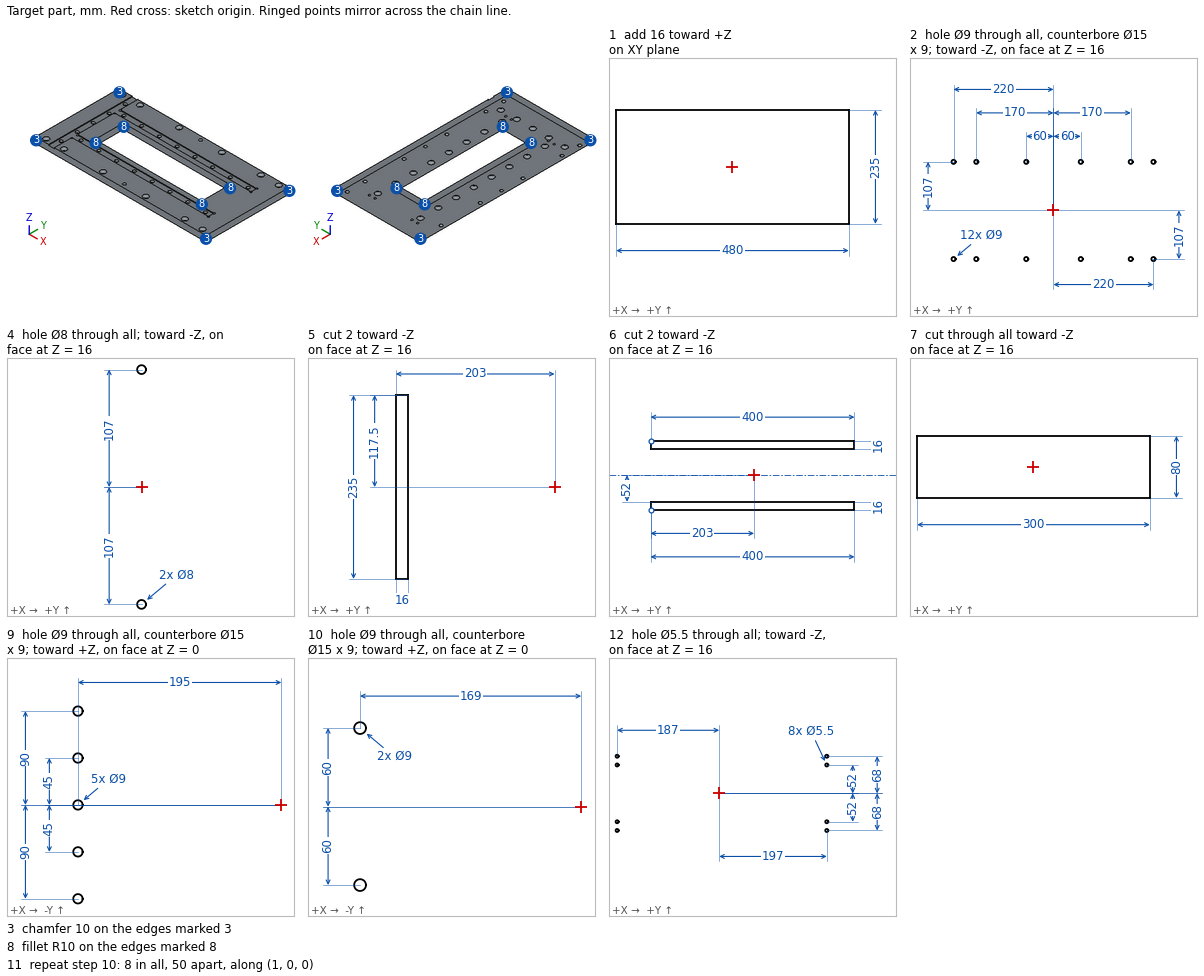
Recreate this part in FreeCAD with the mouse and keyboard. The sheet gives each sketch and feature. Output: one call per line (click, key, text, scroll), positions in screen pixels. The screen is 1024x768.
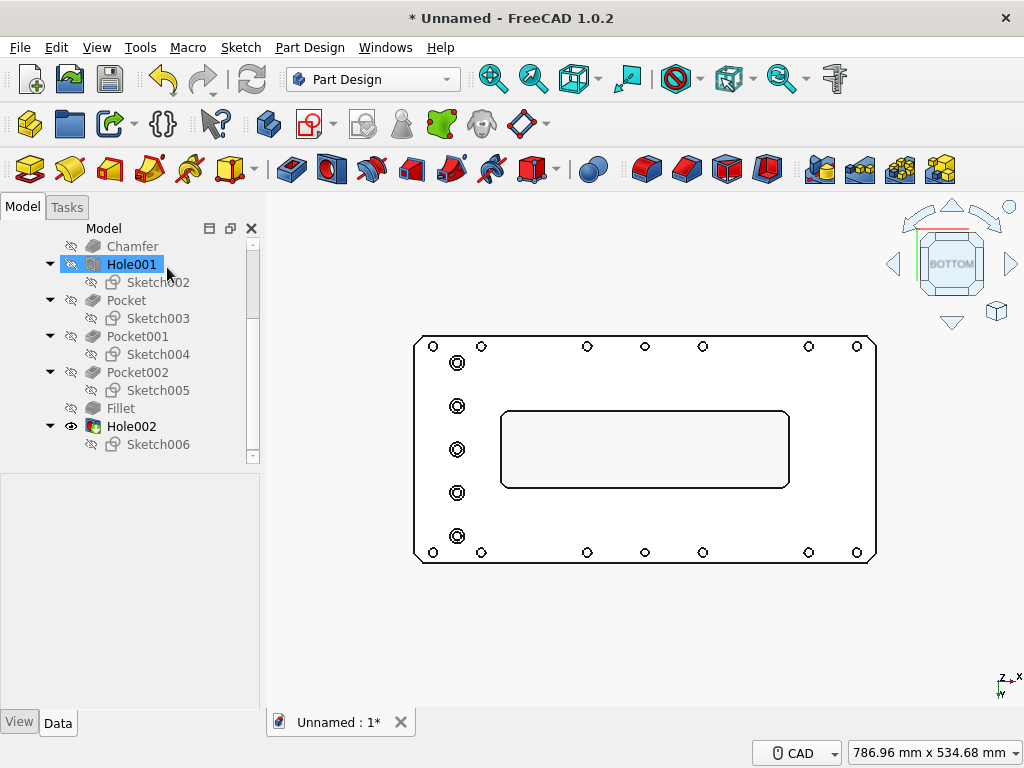
click(843, 513)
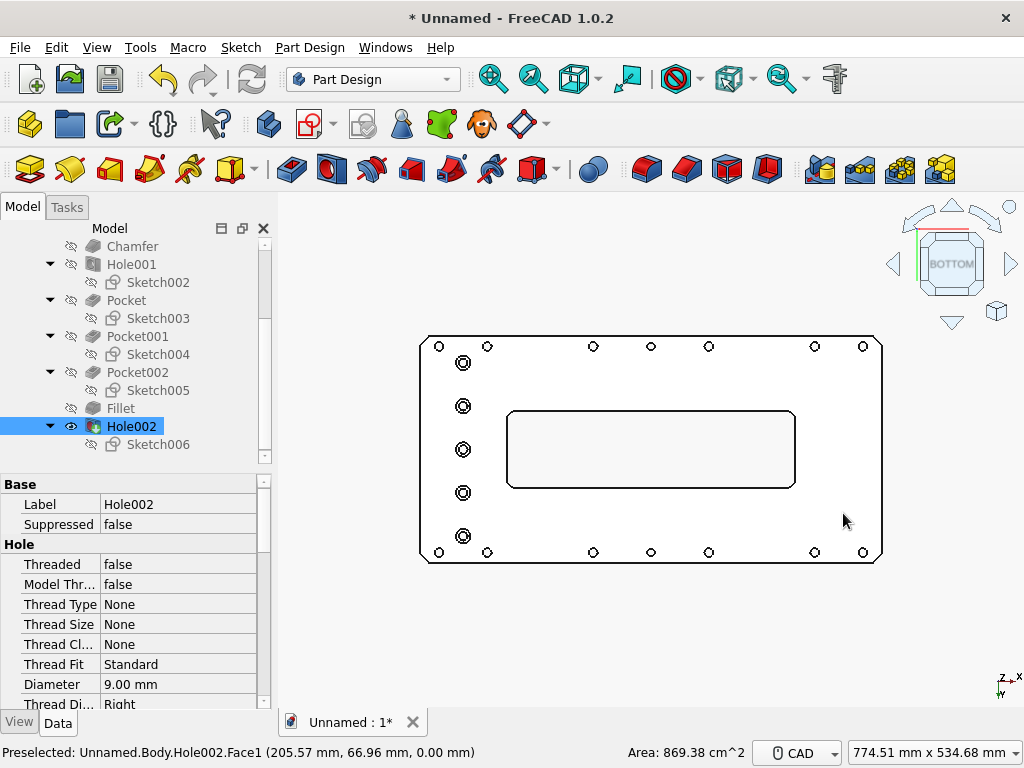
click(310, 124)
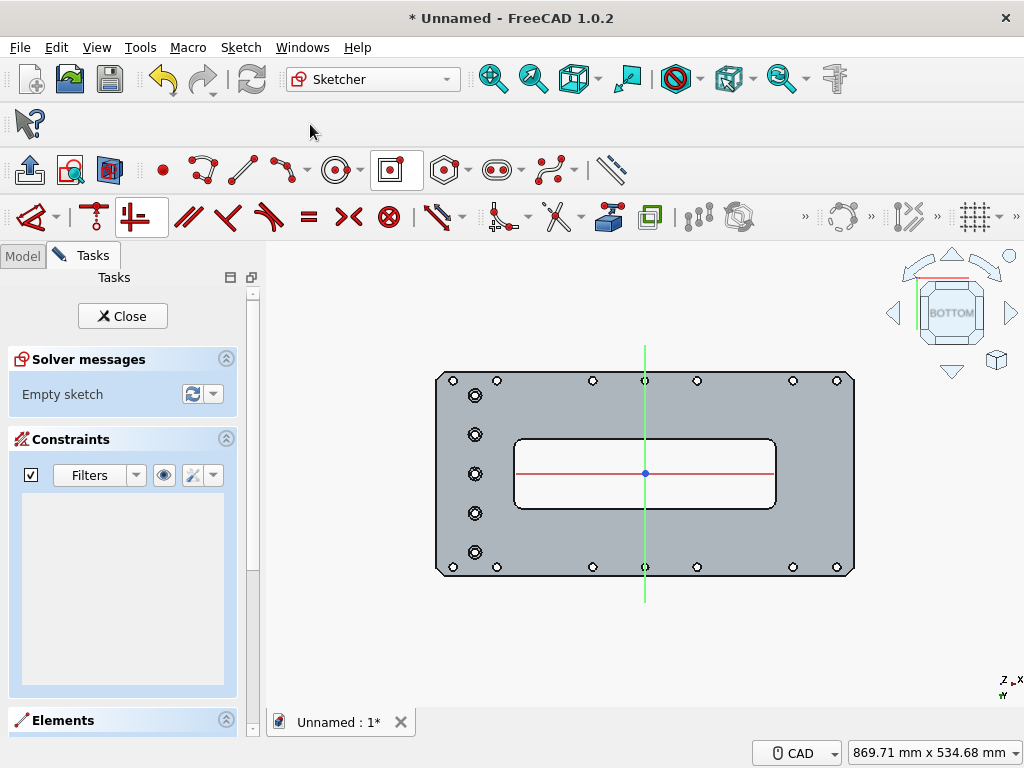
scroll(565, 474, up, 5)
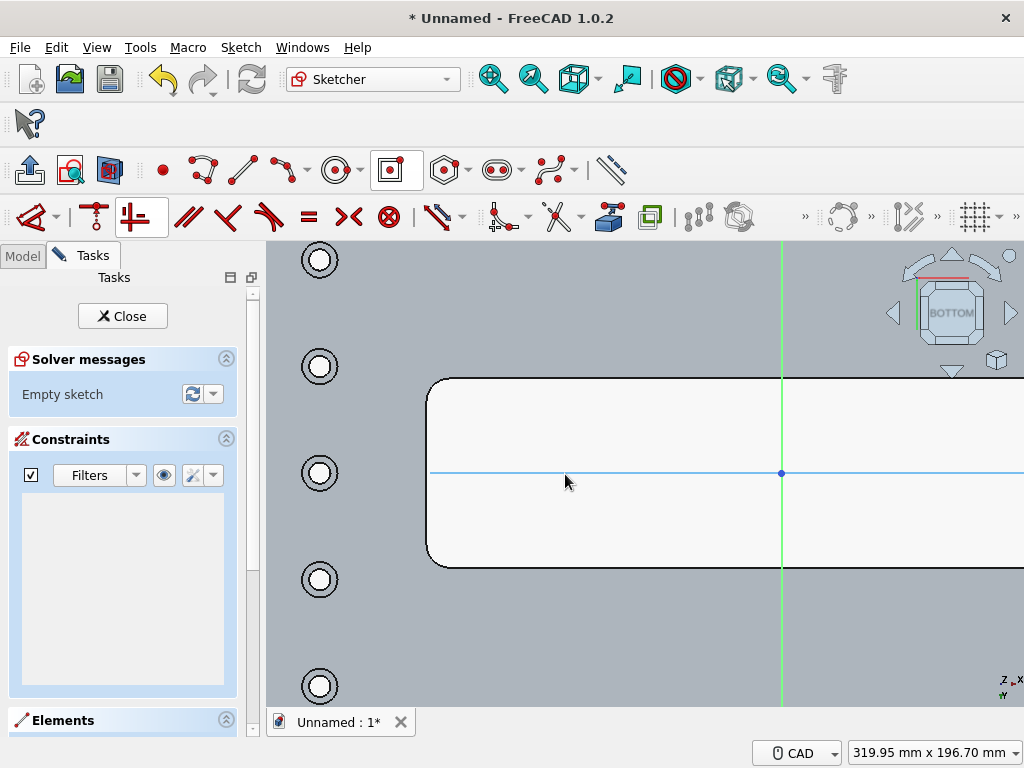
click(336, 170)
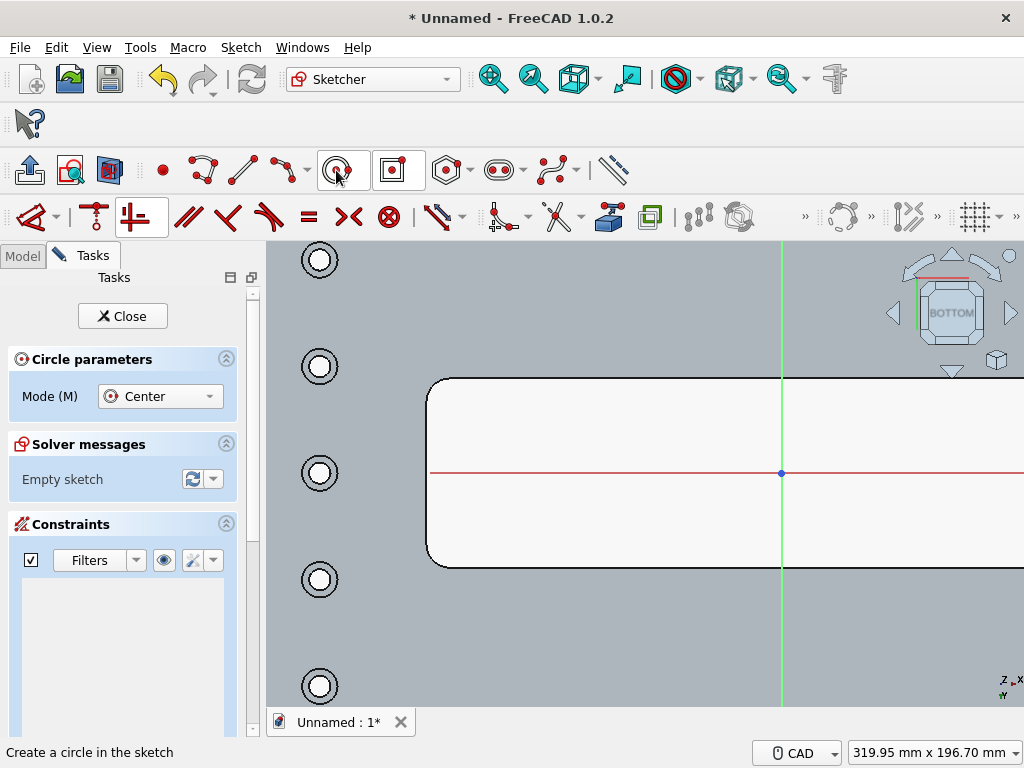
scroll(381, 331, up, 4)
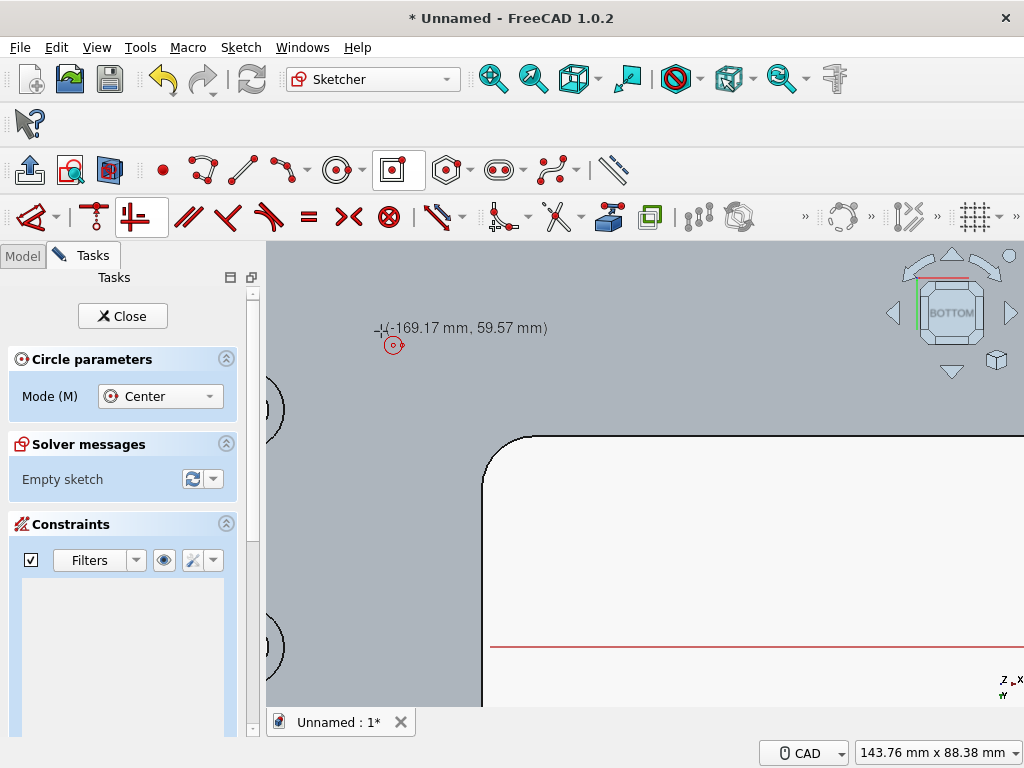
click(382, 331)
move(398, 314)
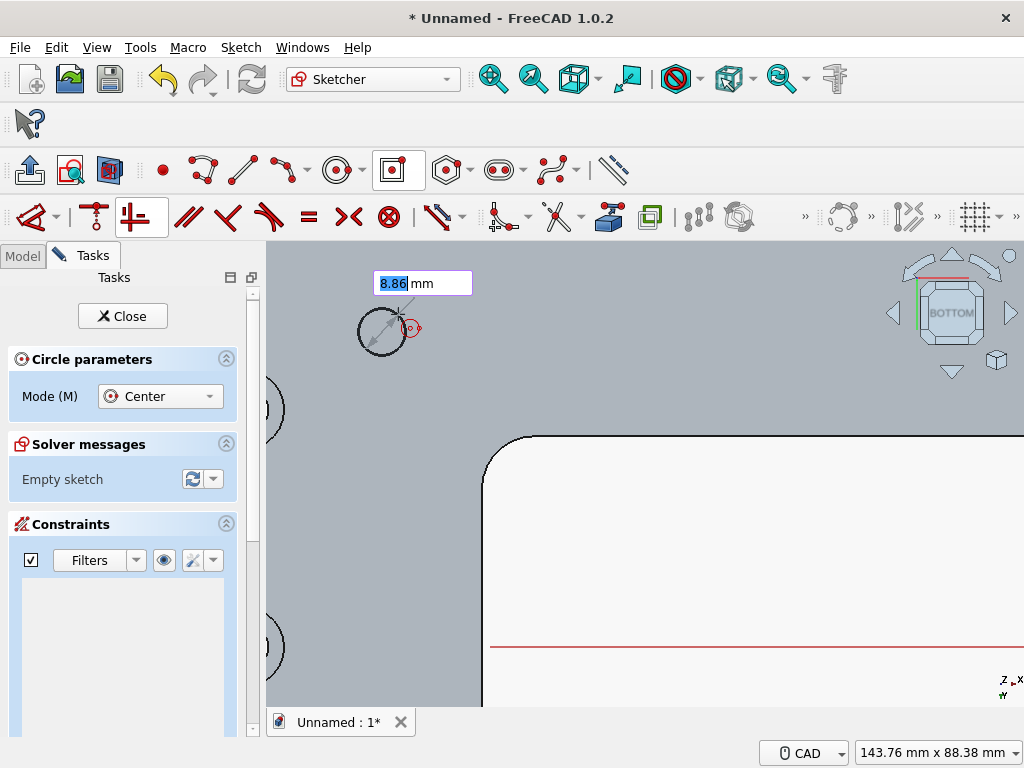
text(9)
key(Return)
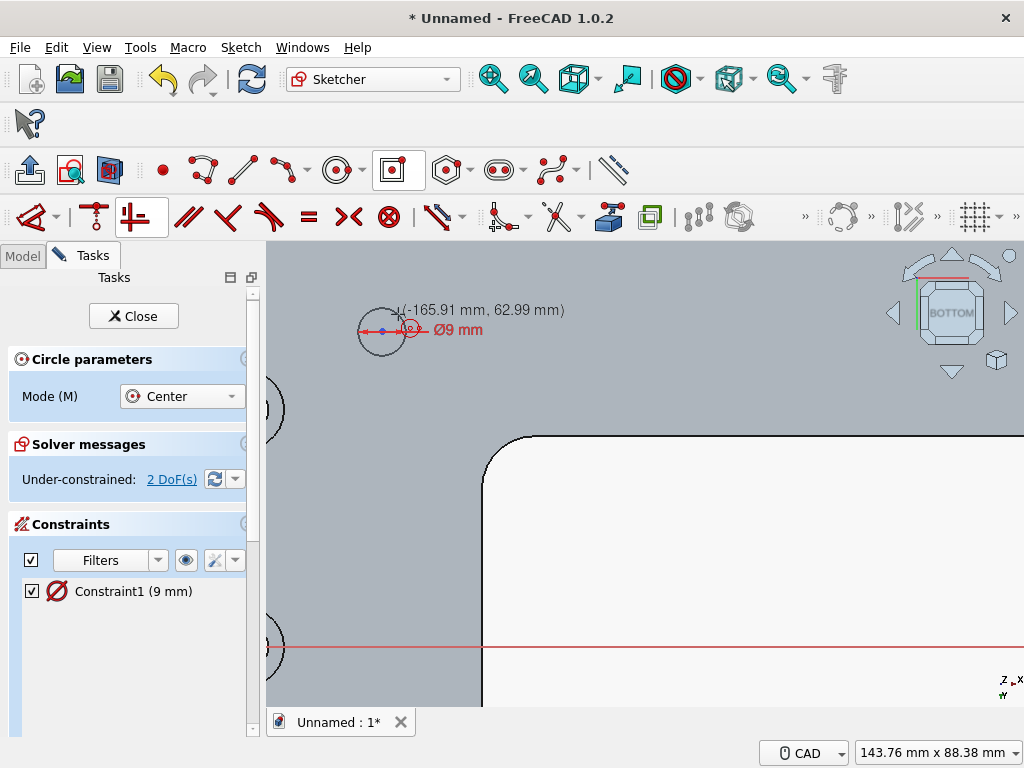
scroll(382, 333, down, 4)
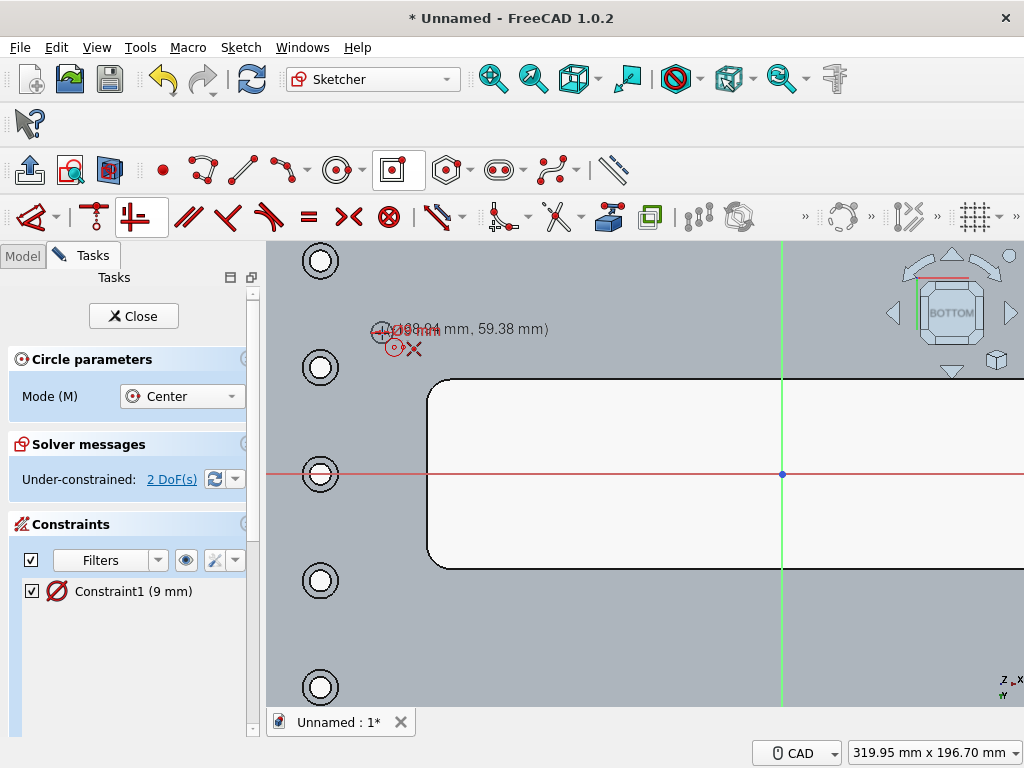
scroll(382, 616, up, 4)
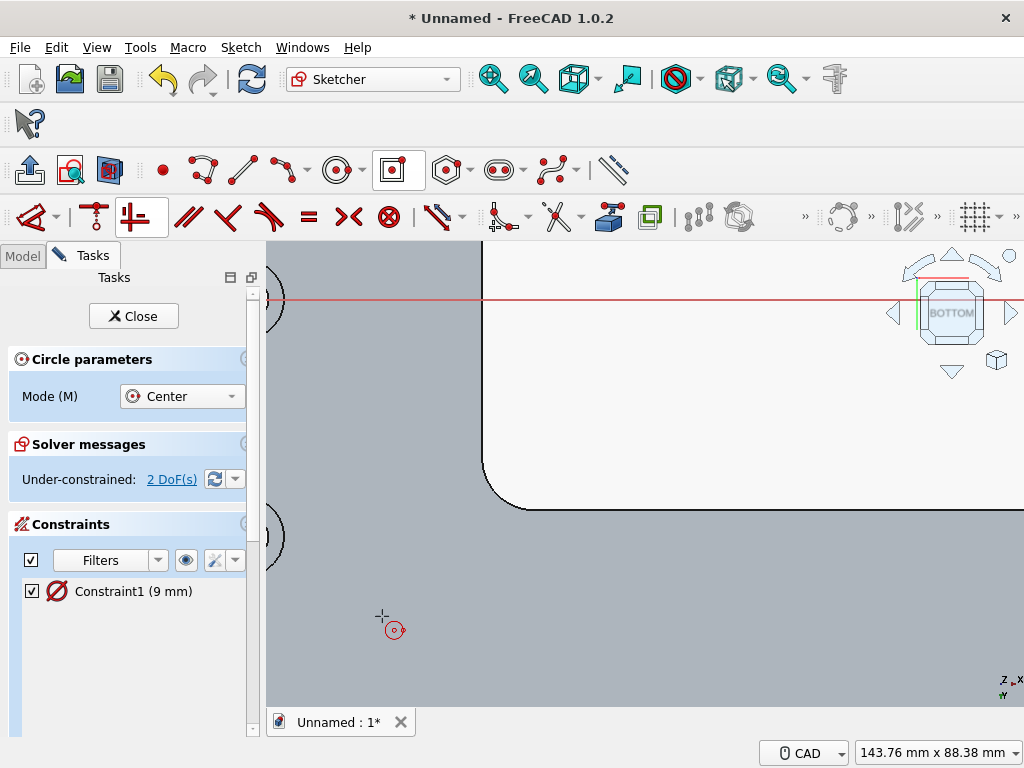
click(382, 616)
move(398, 599)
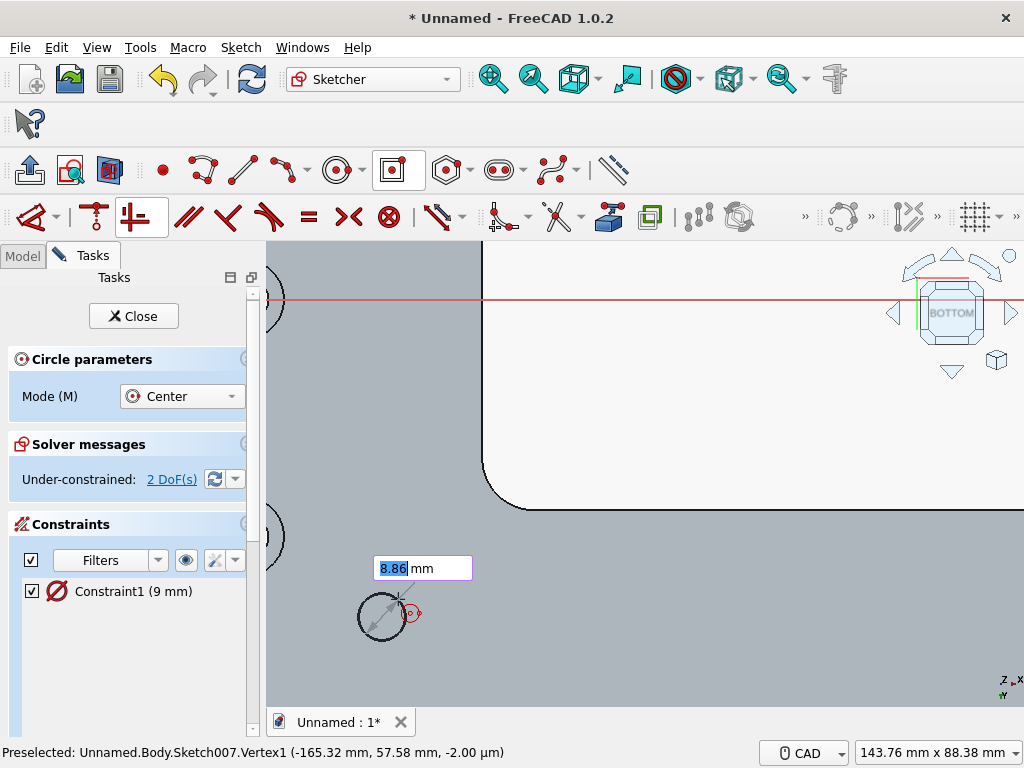
text(9)
key(Return)
key(Escape)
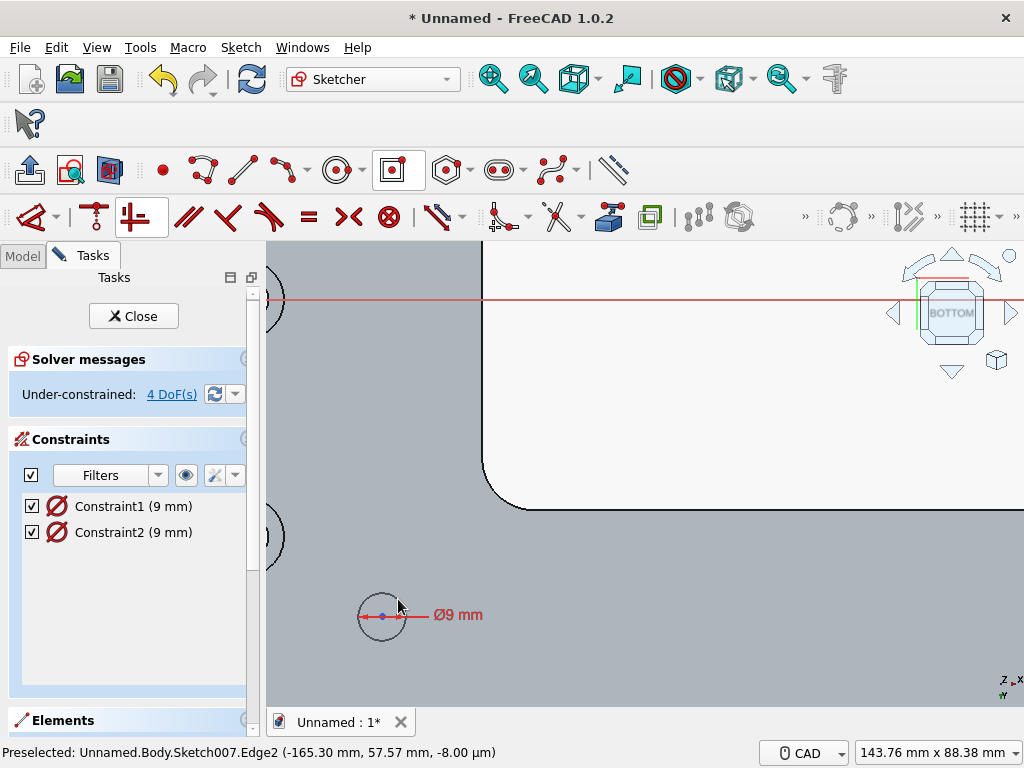
scroll(382, 616, down, 4)